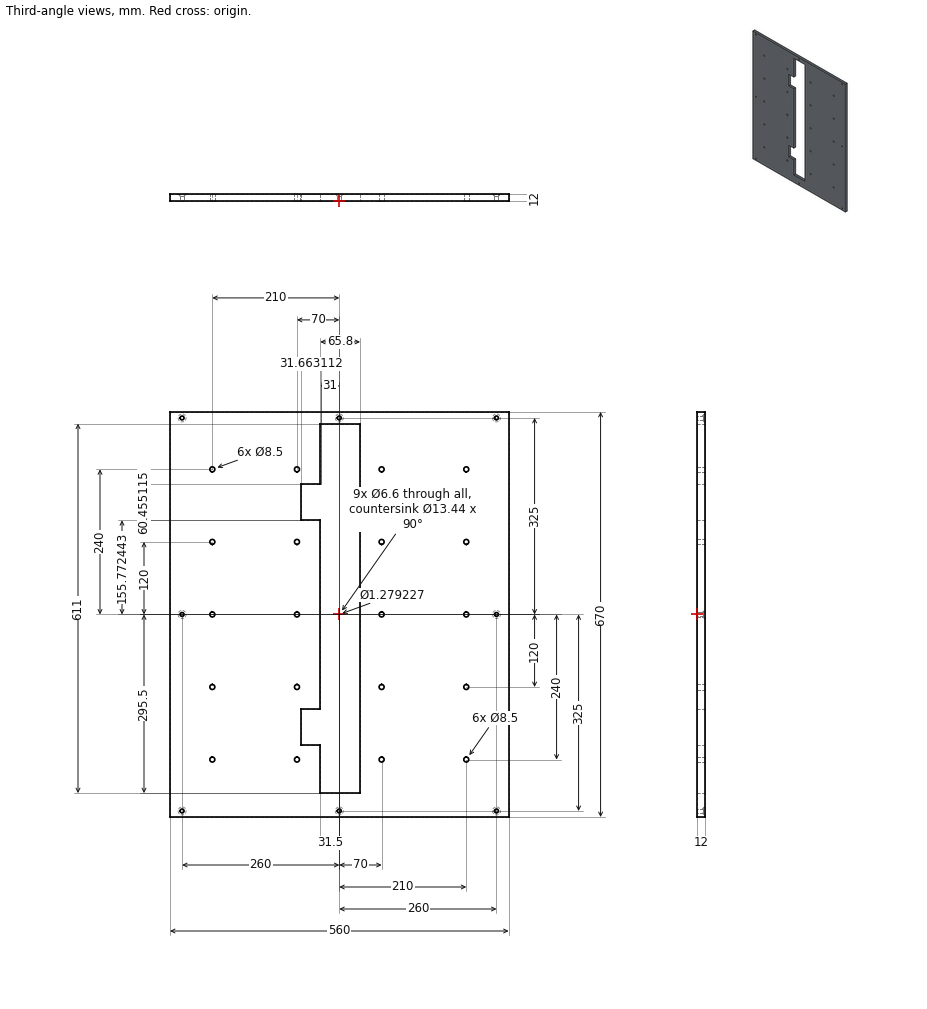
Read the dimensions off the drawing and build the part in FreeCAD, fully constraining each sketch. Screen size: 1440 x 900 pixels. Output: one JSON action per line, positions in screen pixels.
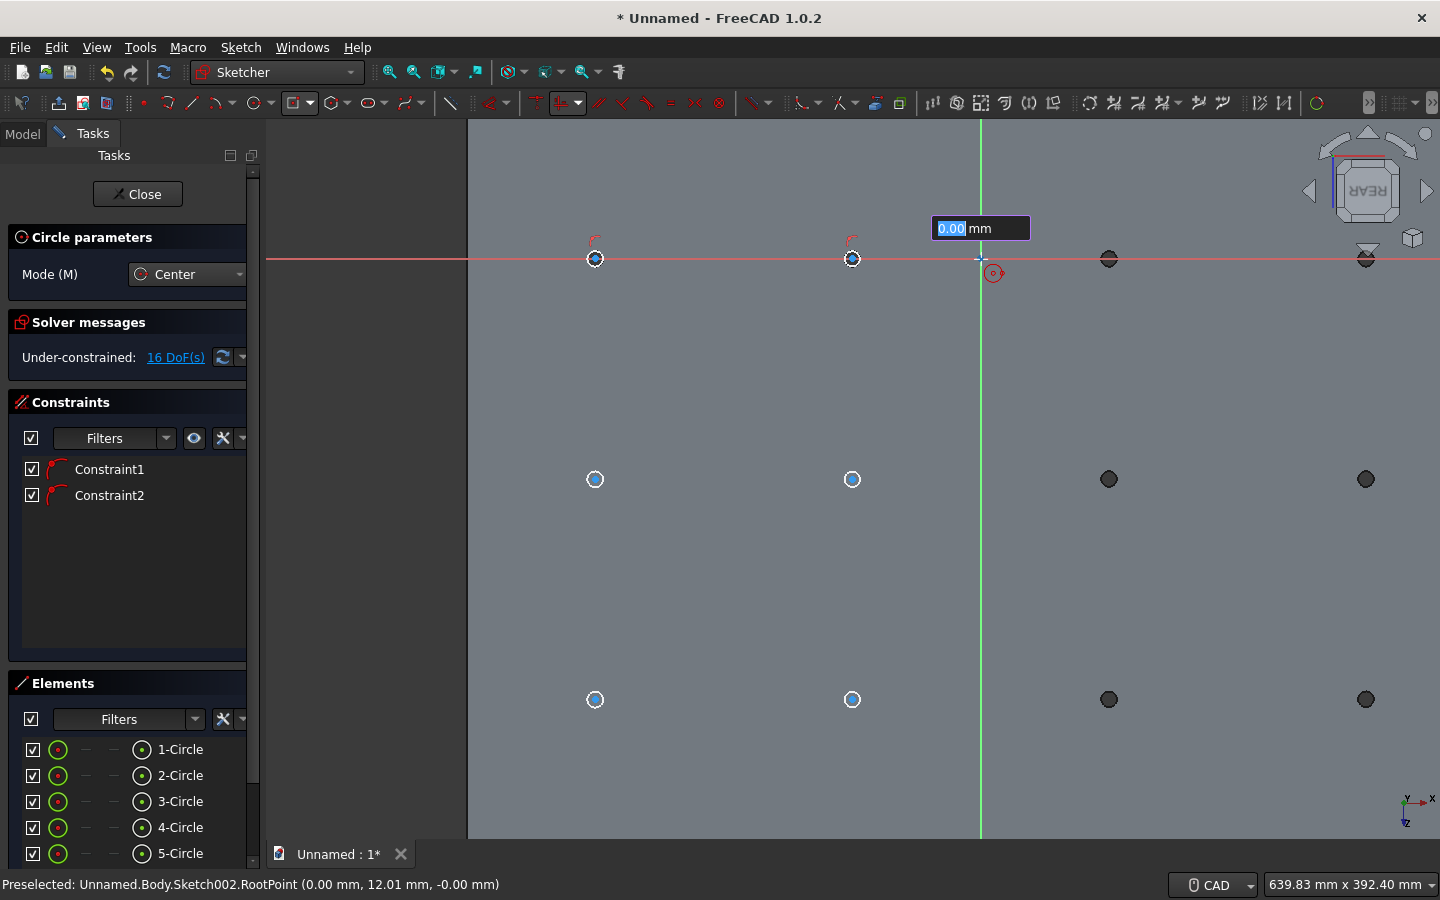
{"action": "scroll", "coordinate": [981, 258], "scroll_direction": "up", "scroll_amount": 15}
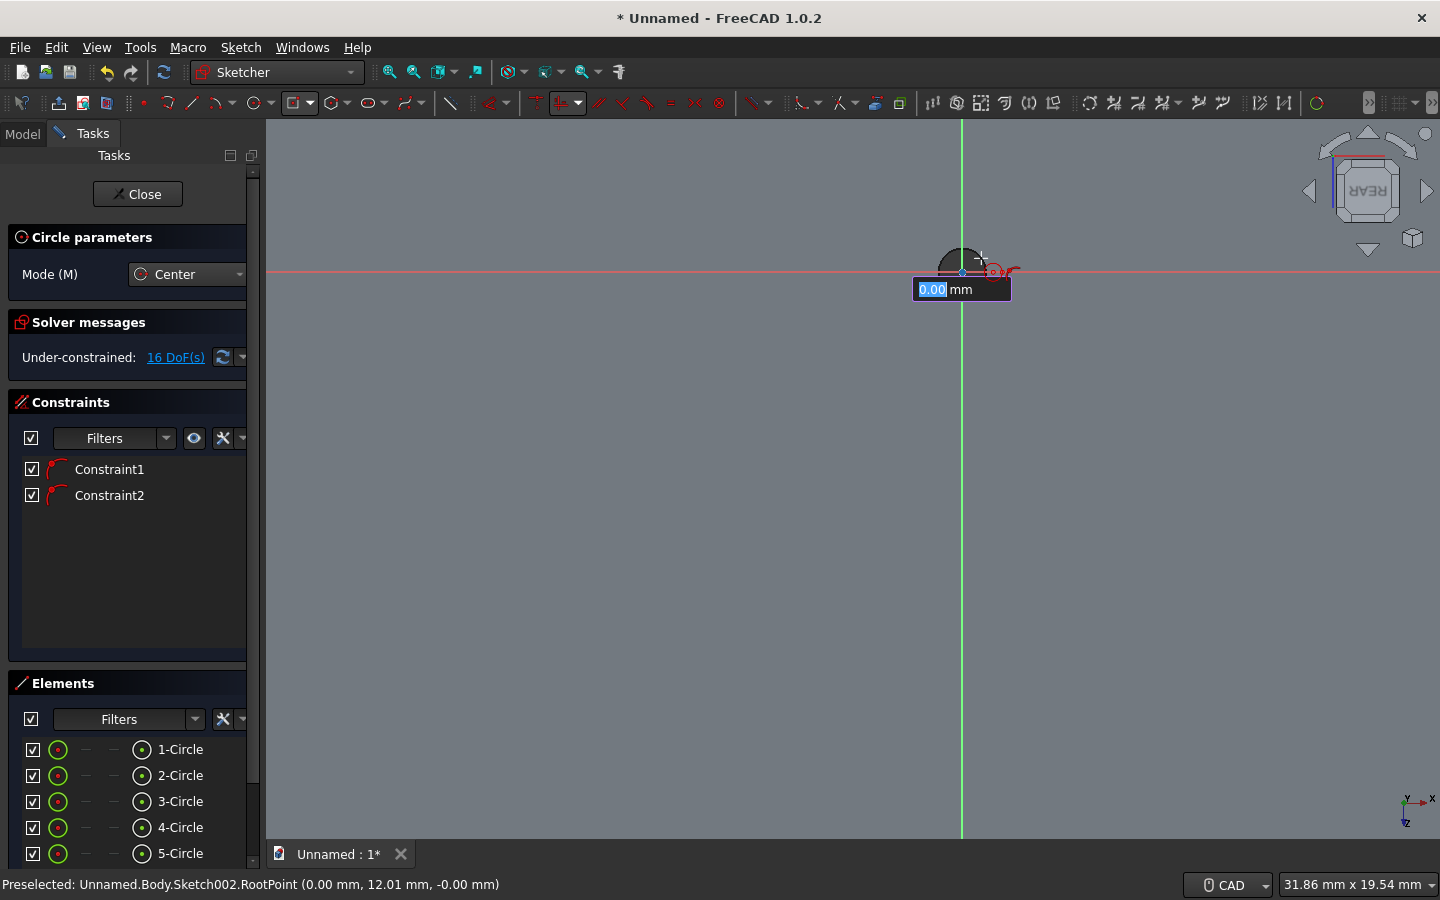
{"action": "left_click", "coordinate": [979, 255]}
{"action": "key", "text": "Escape"}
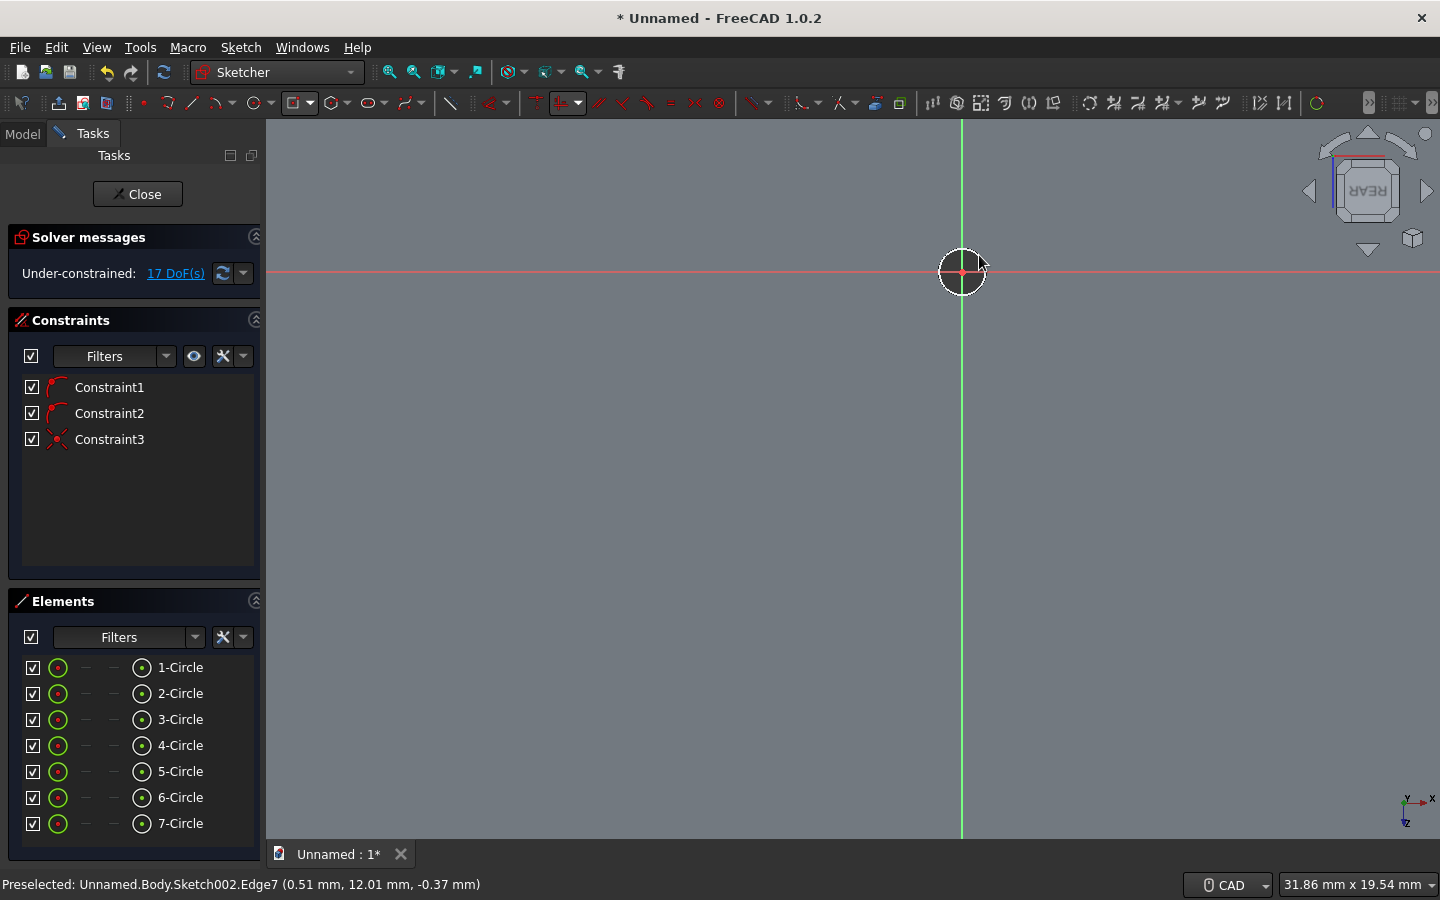
{"action": "scroll", "coordinate": [981, 258], "scroll_direction": "down", "scroll_amount": 15}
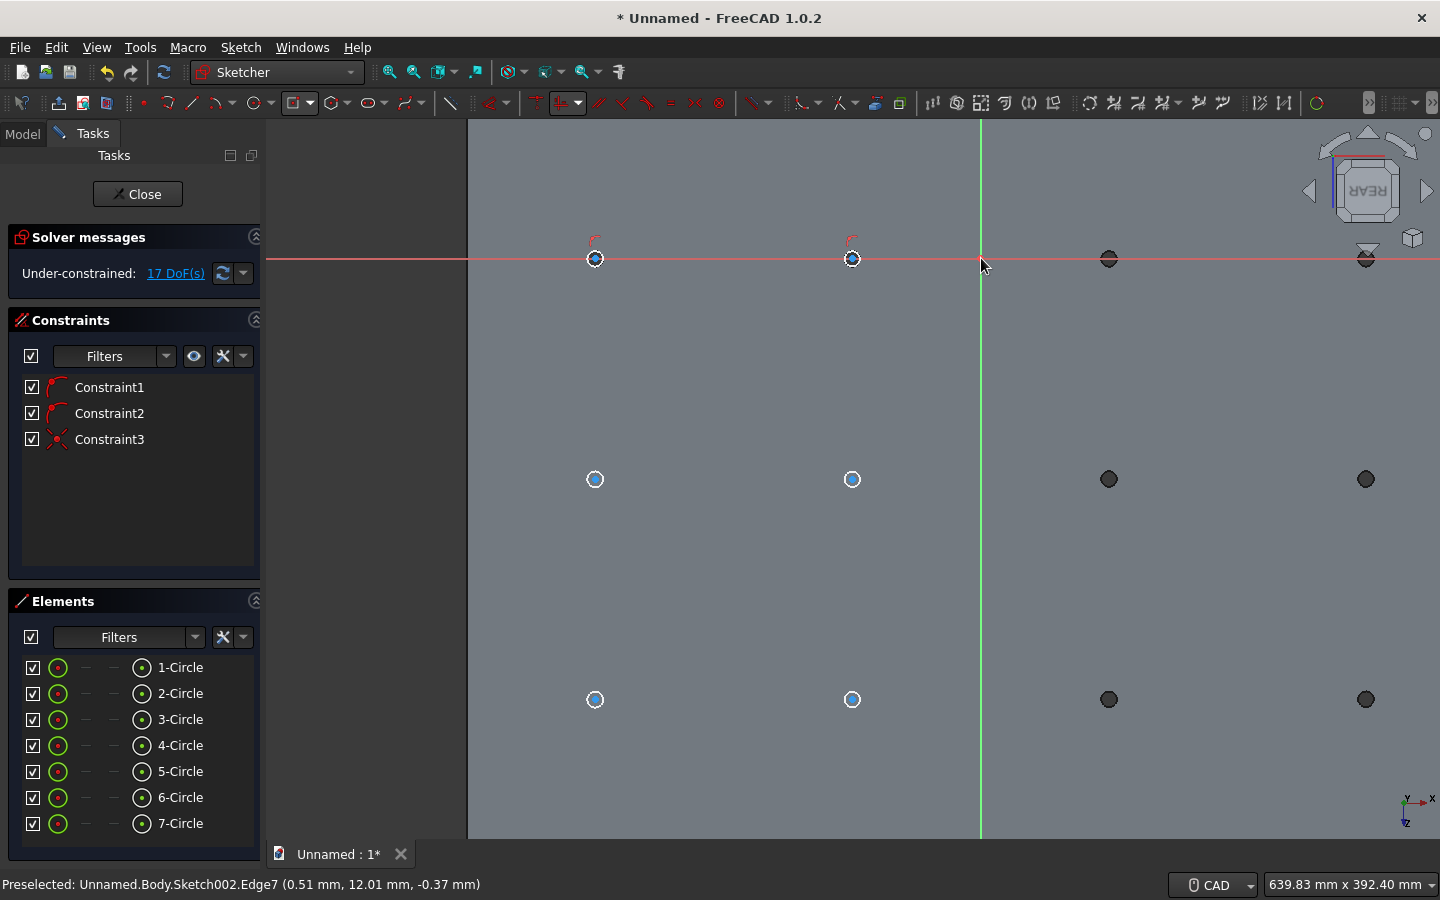
{"action": "scroll", "coordinate": [601, 694], "scroll_direction": "up", "scroll_amount": 3}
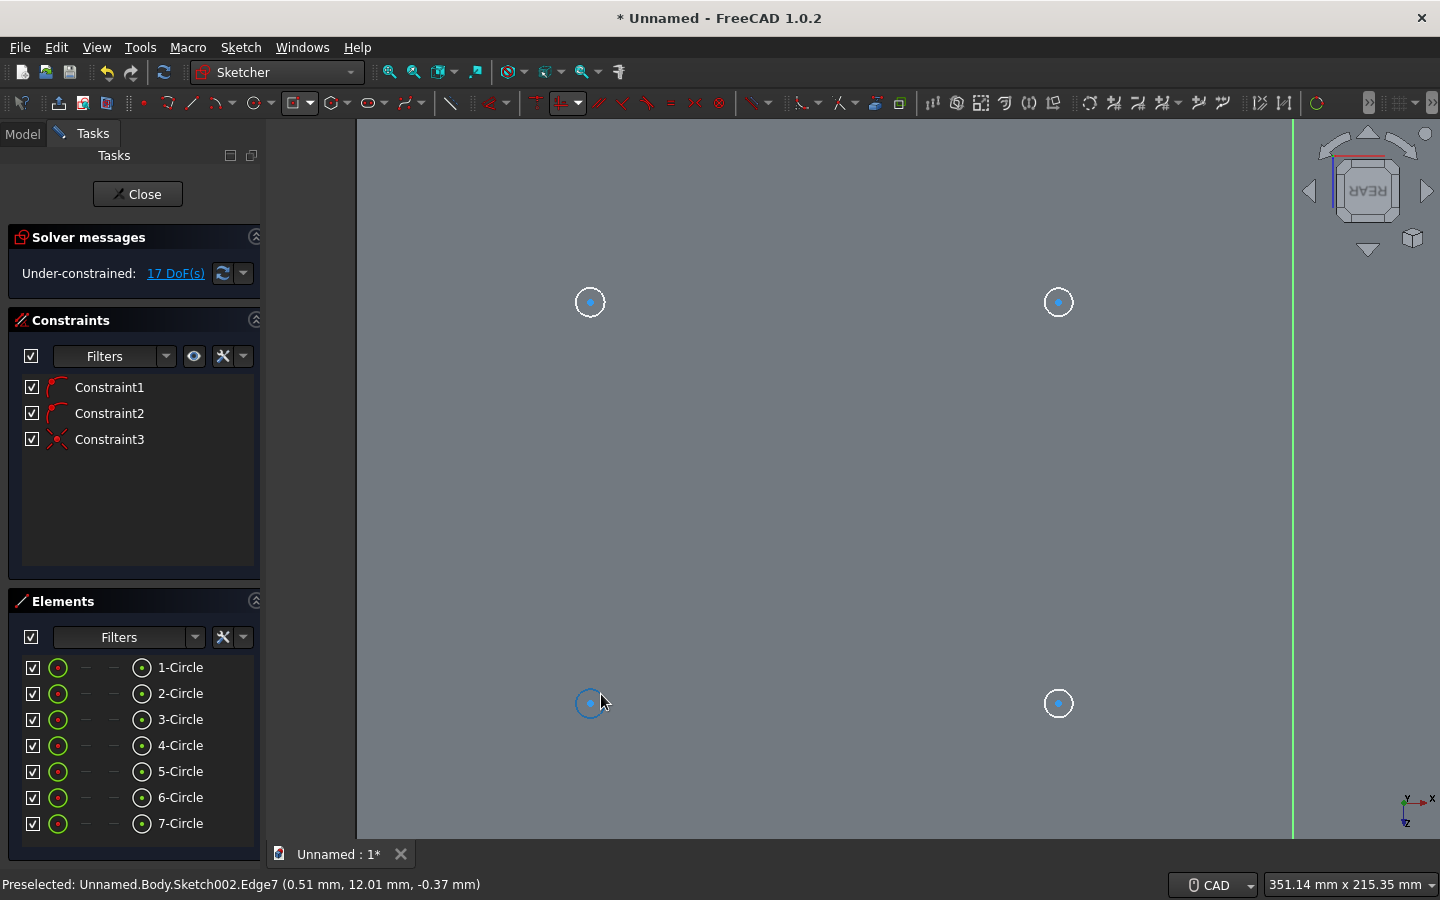
{"action": "left_click", "coordinate": [600, 693]}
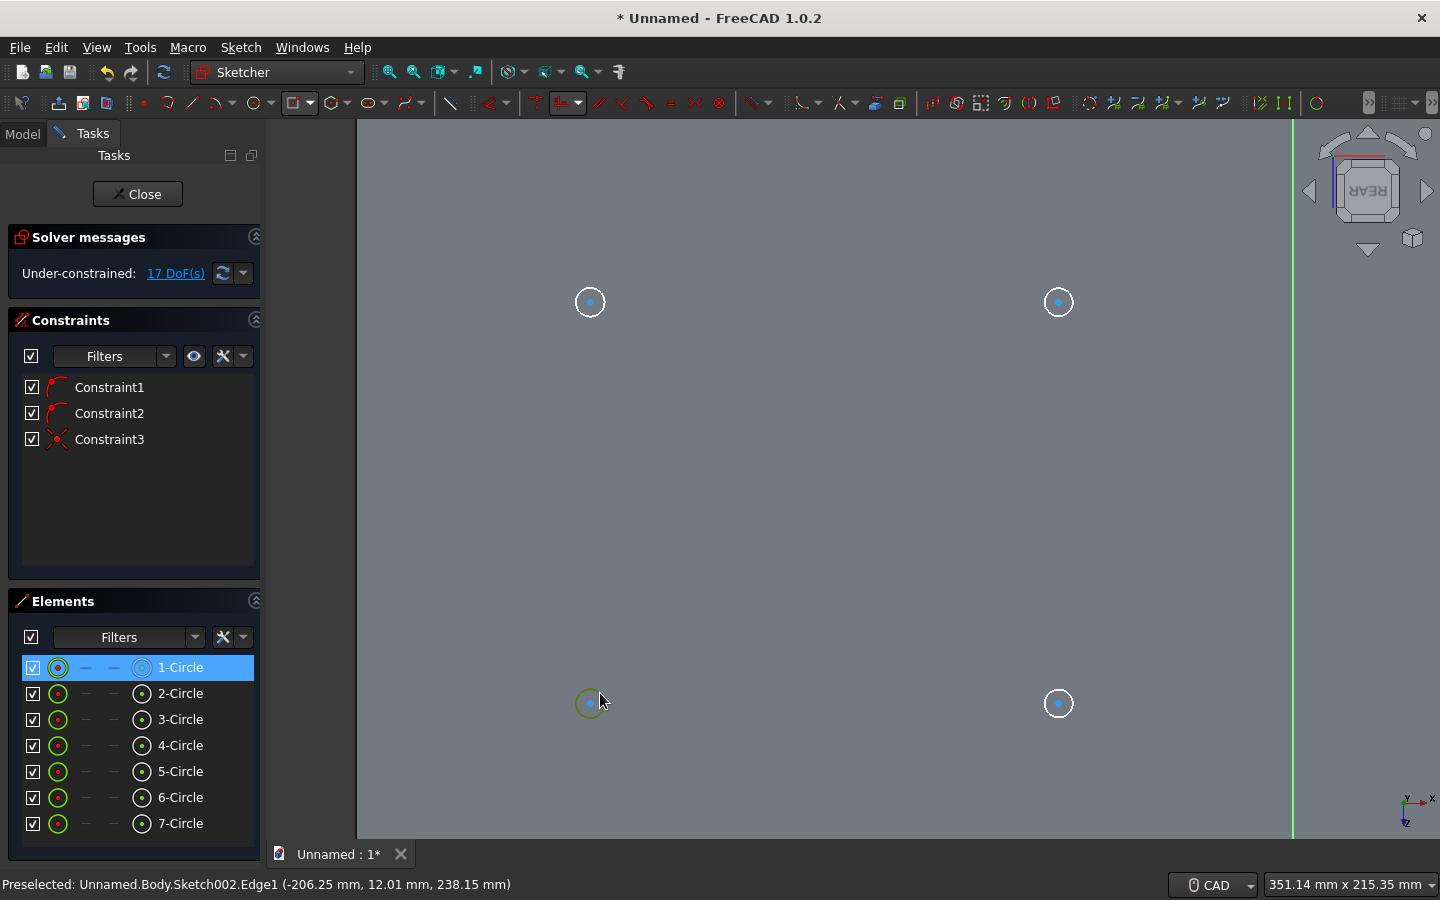
{"action": "left_click", "coordinate": [1069, 694]}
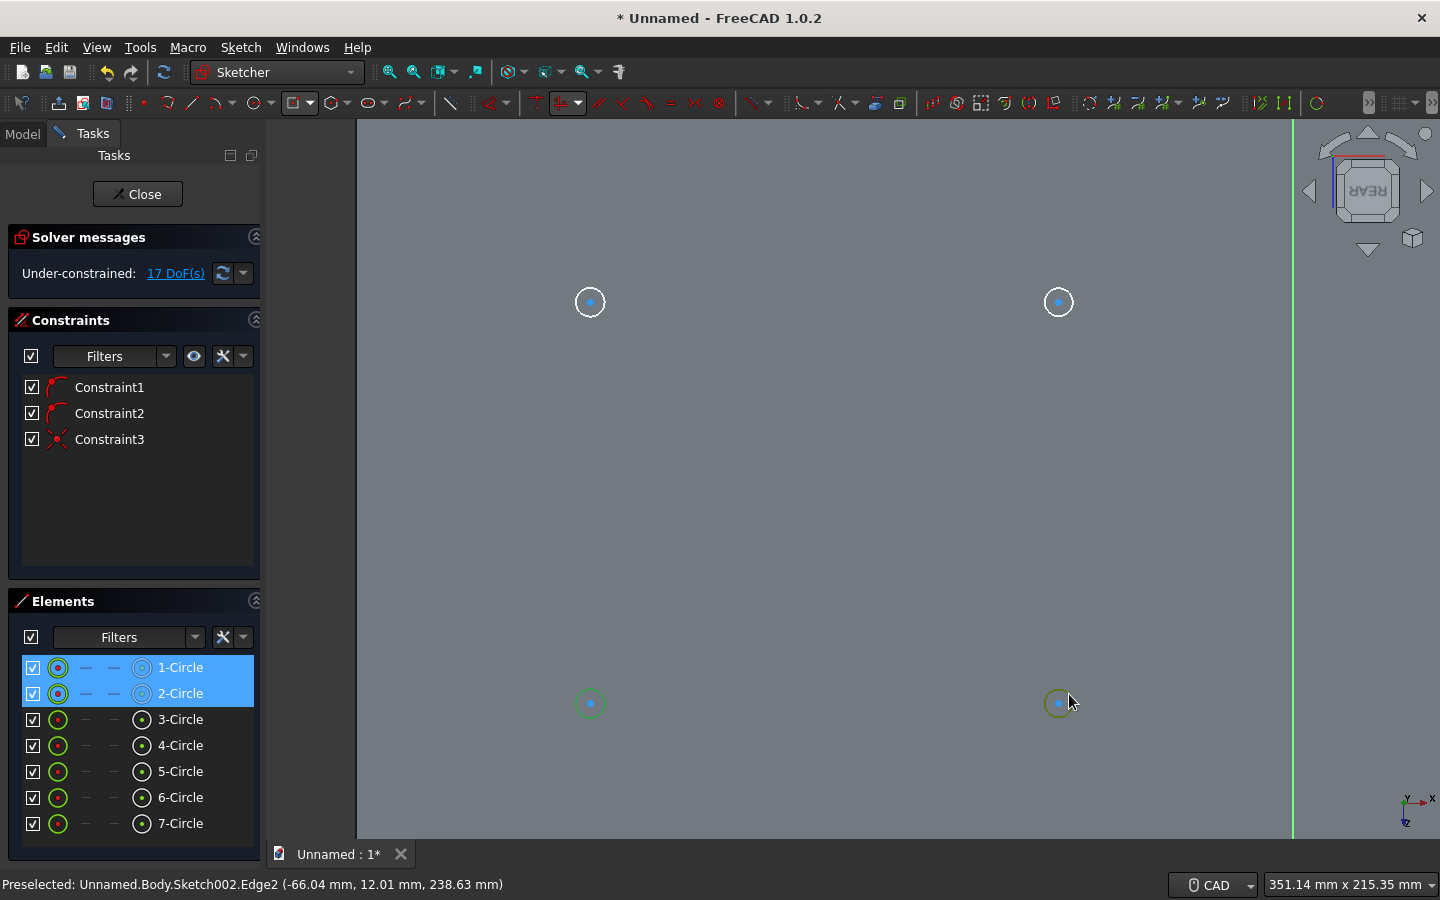
{"action": "left_click", "coordinate": [600, 292]}